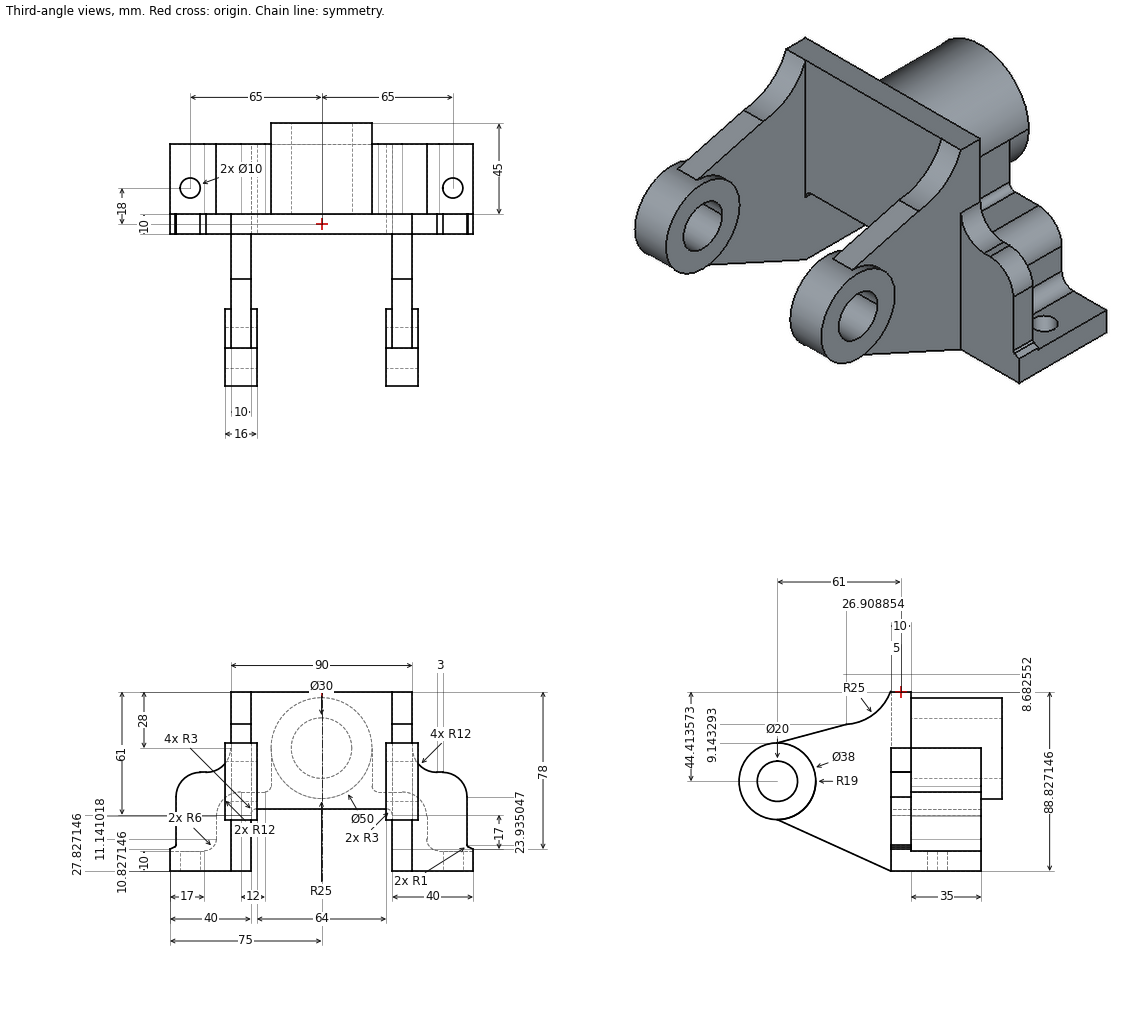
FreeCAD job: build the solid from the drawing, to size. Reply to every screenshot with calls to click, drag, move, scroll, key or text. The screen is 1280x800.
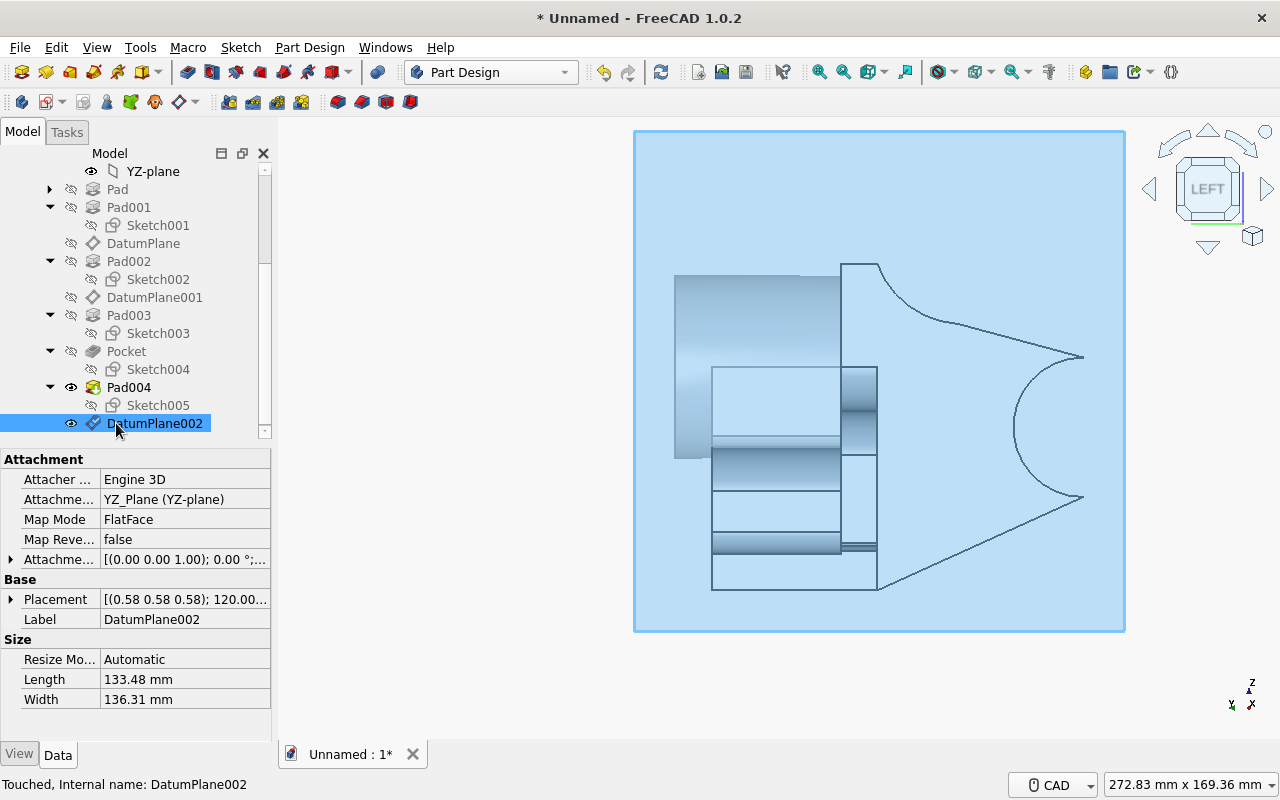
click(46, 102)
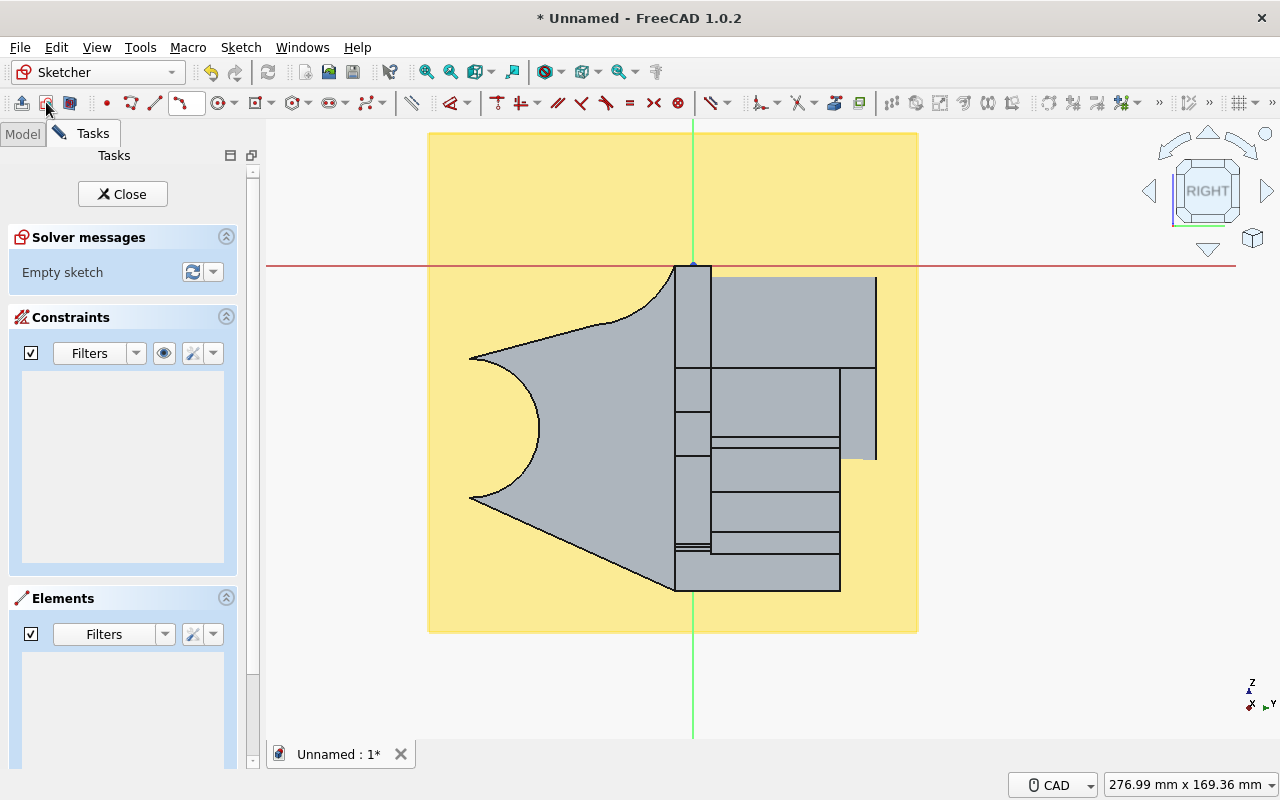
key(q)
key(s)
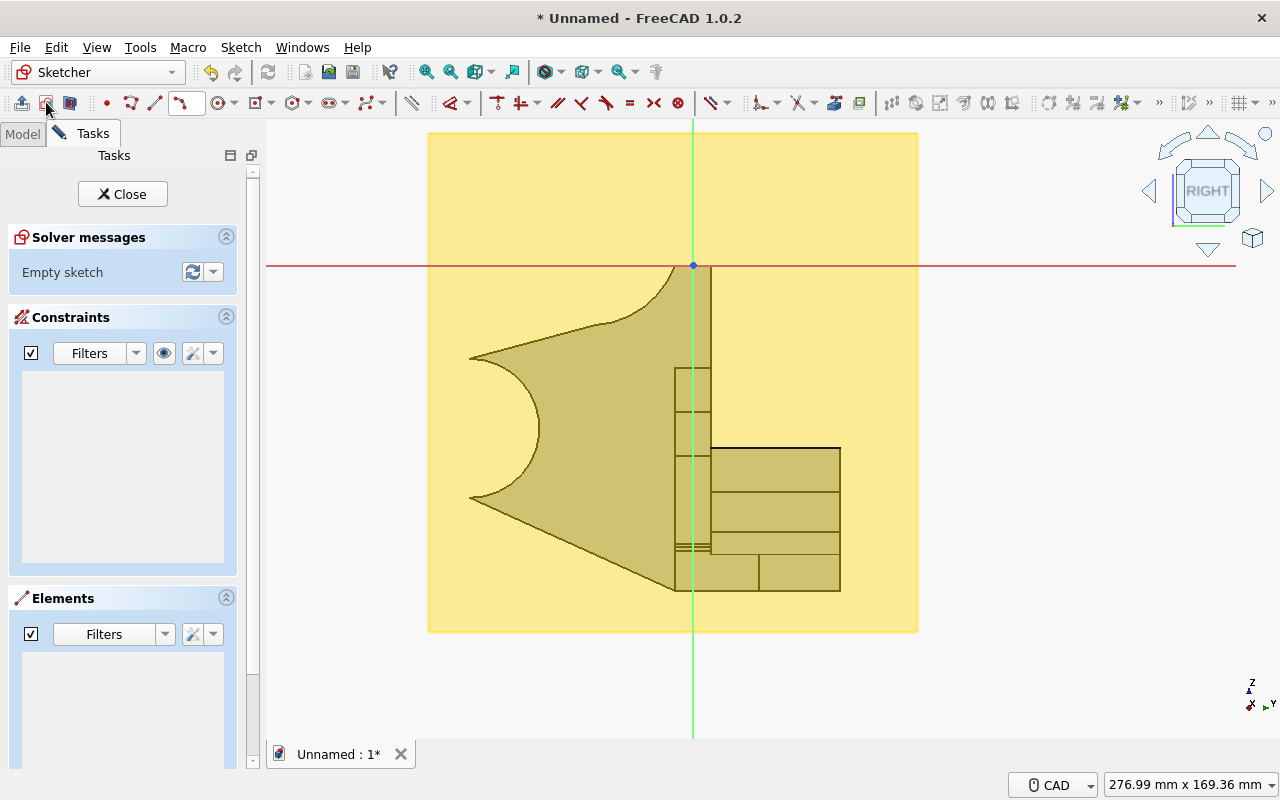
scroll(355, 324, up, 3)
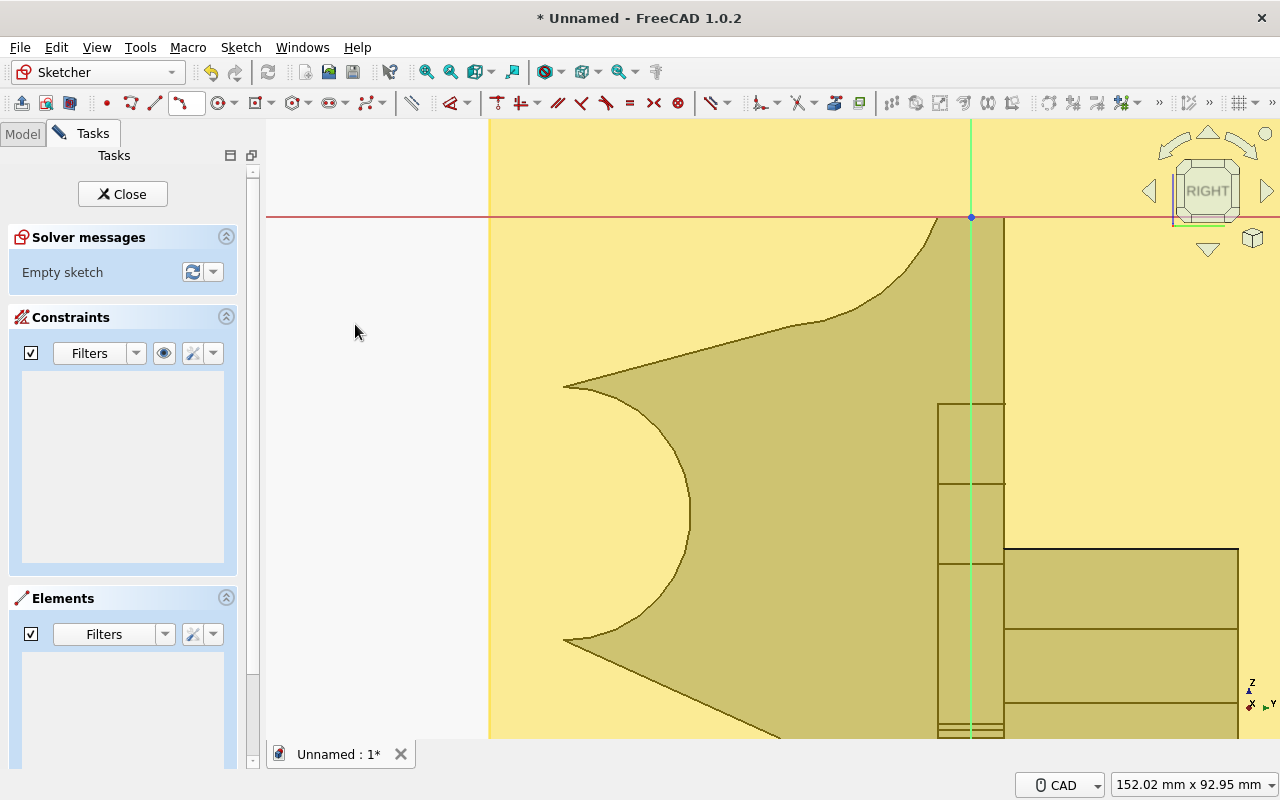
key(g)
key(c)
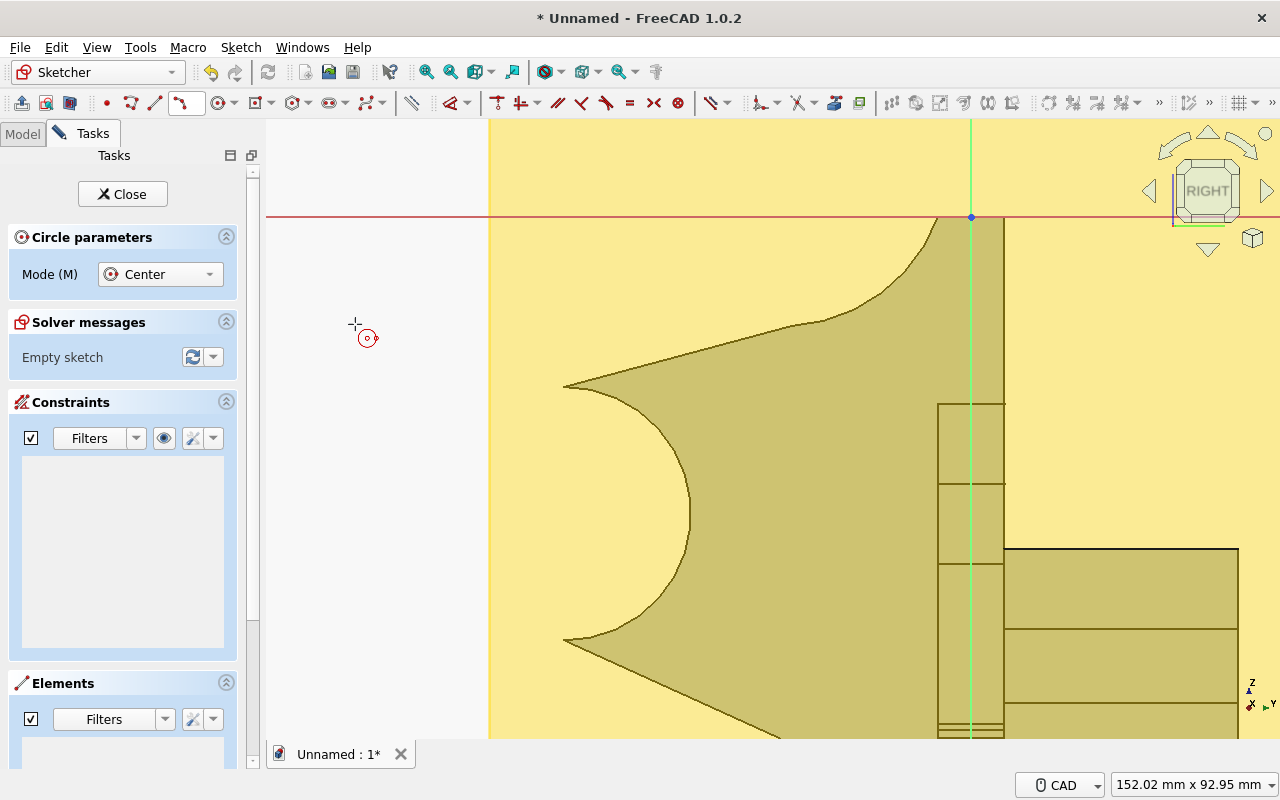
click(564, 514)
click(654, 424)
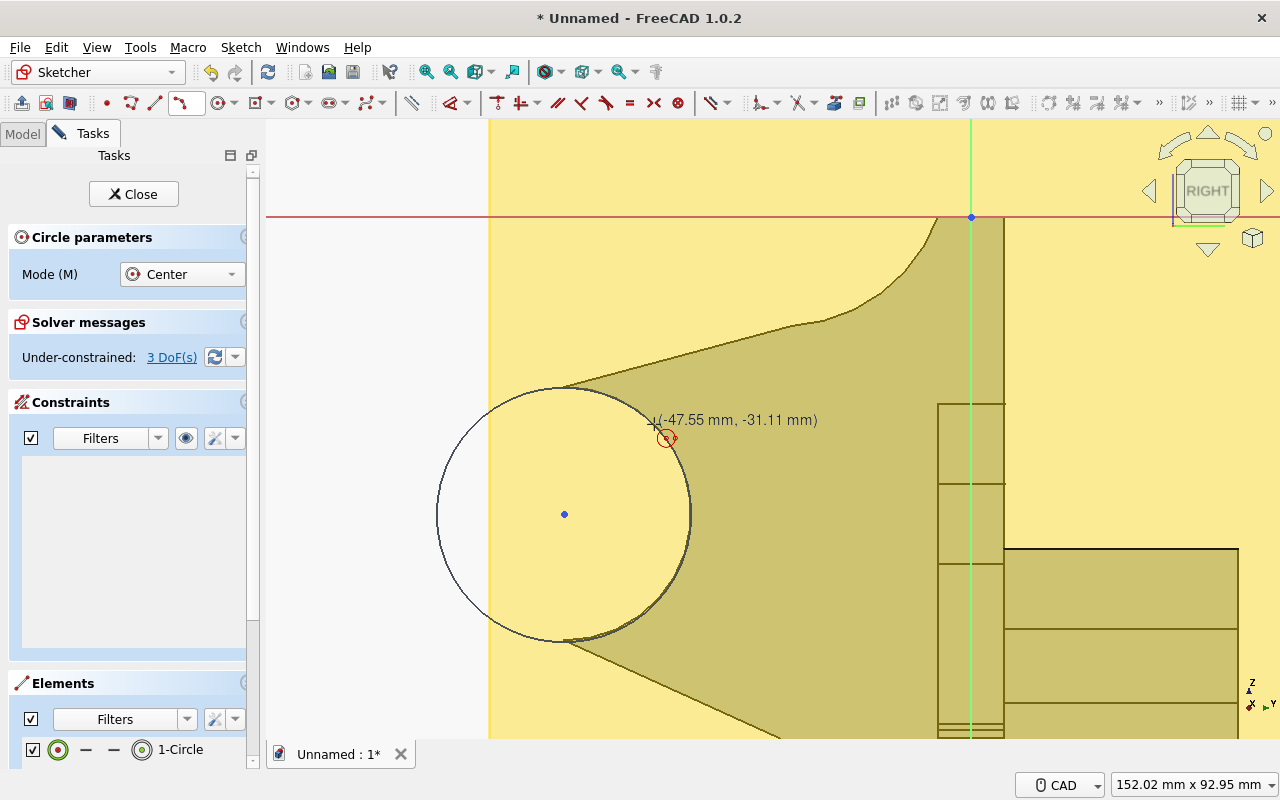
click(564, 515)
click(611, 467)
key(Escape)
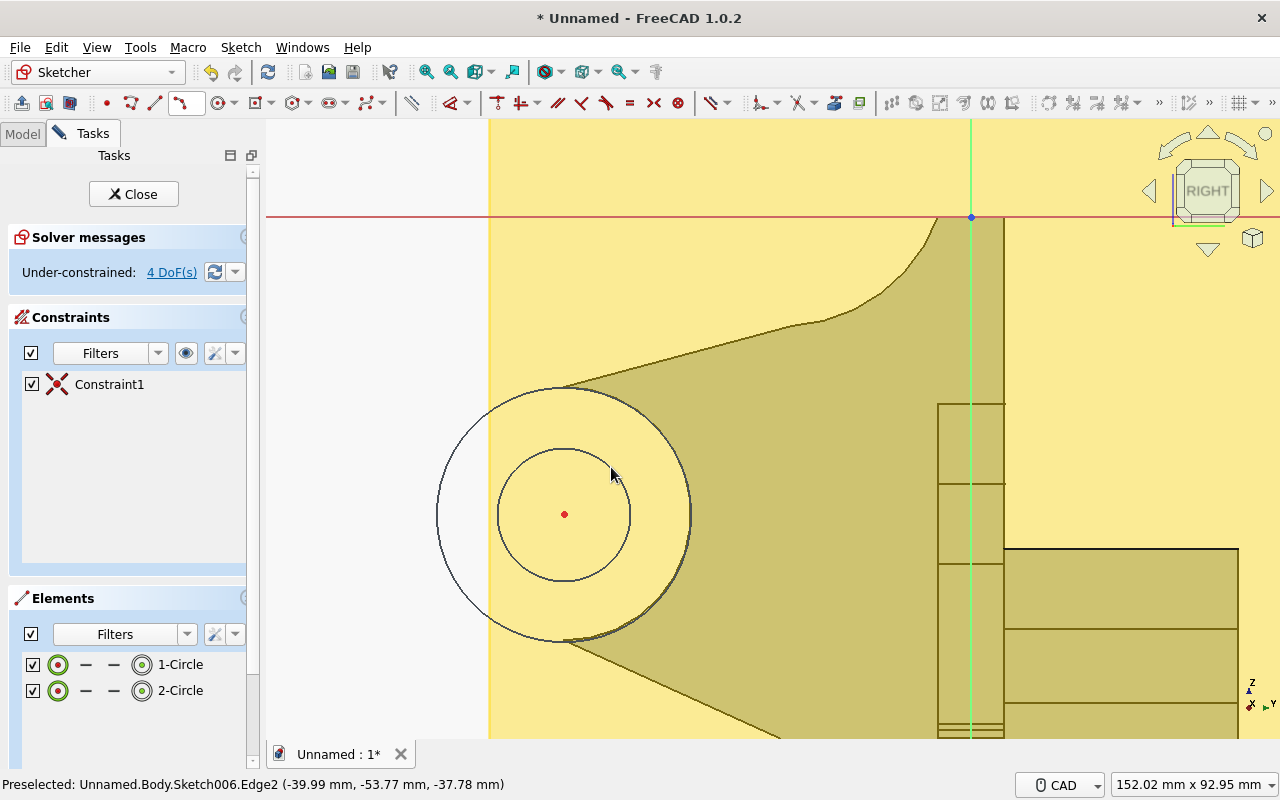
key(d)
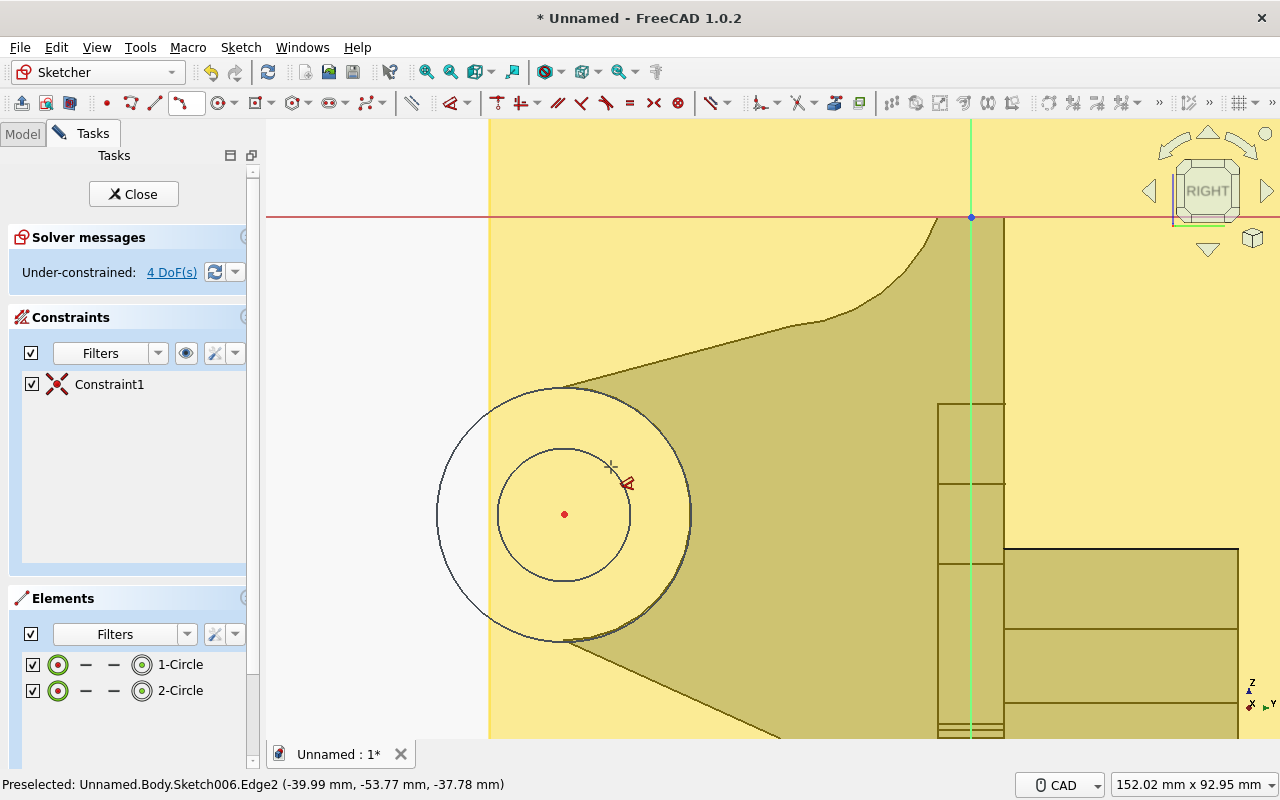
click(654, 425)
click(677, 402)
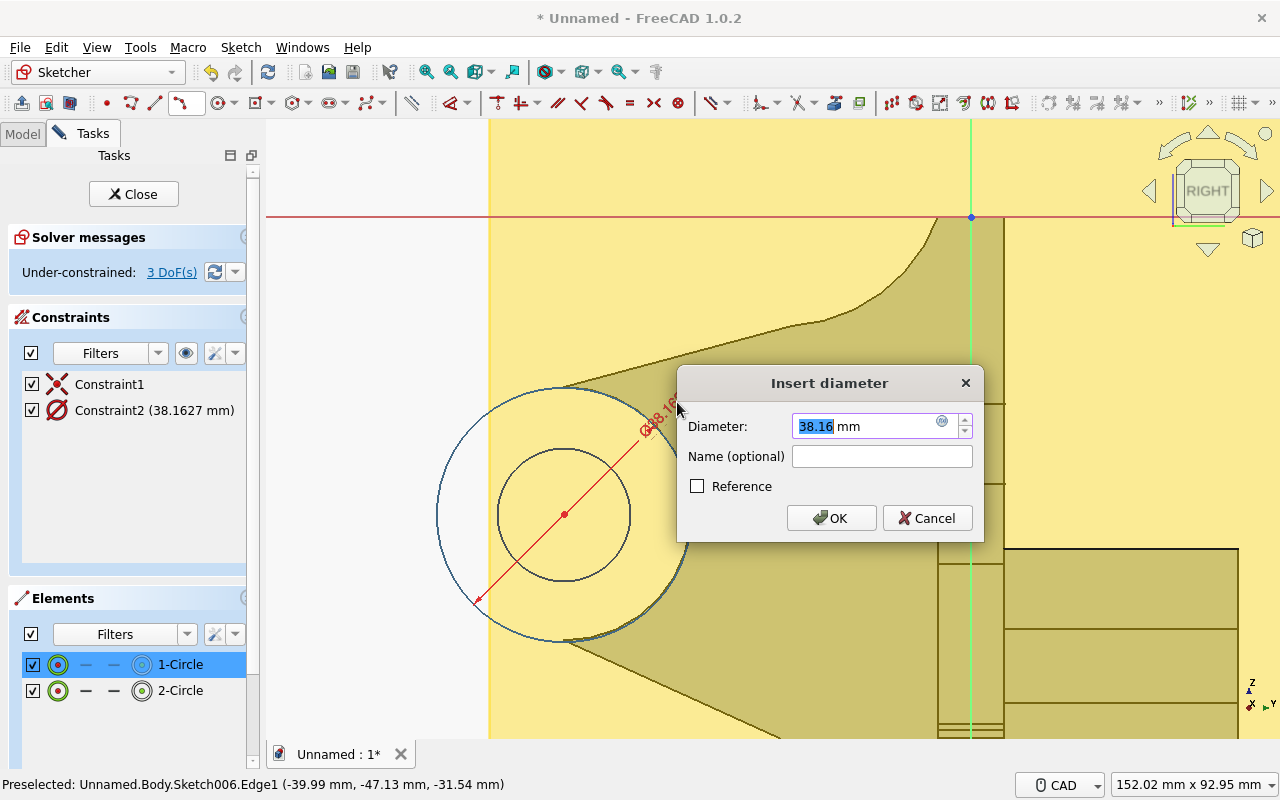
text(38)
key(Return)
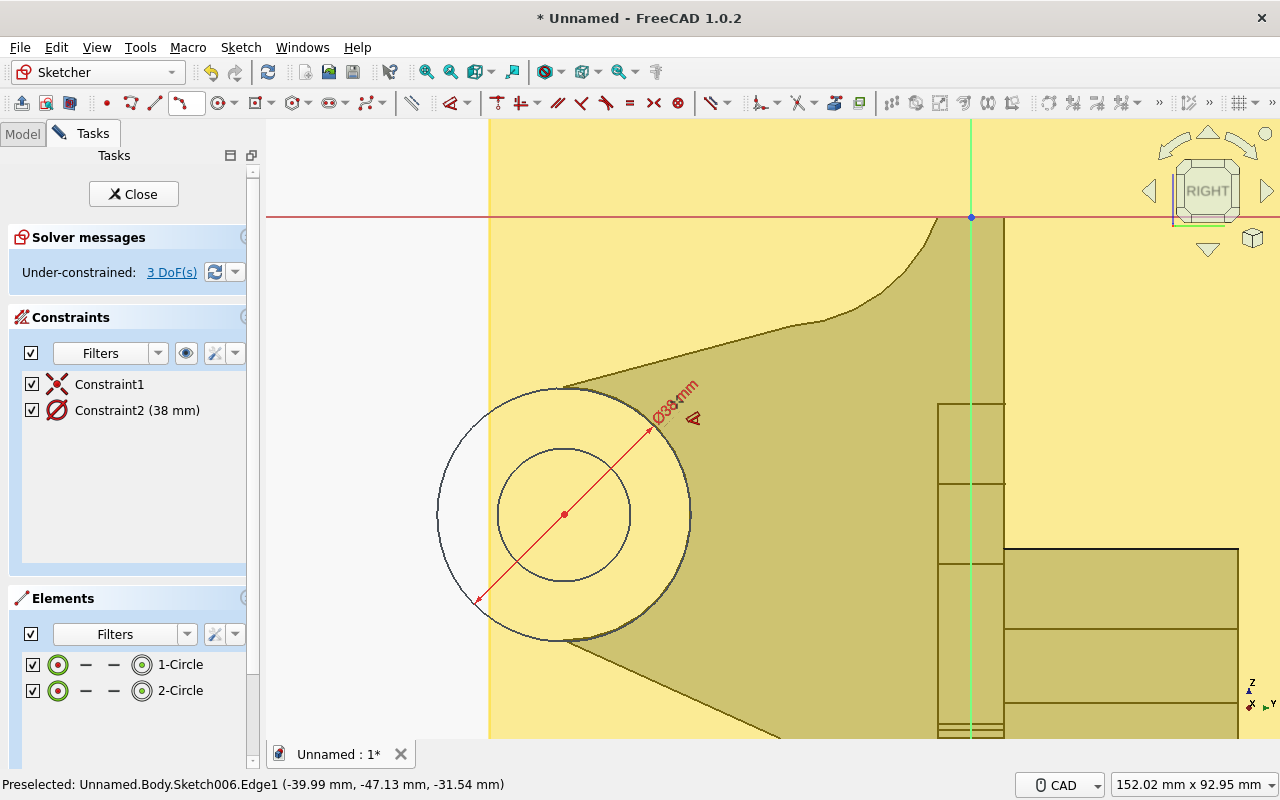
click(611, 468)
click(634, 445)